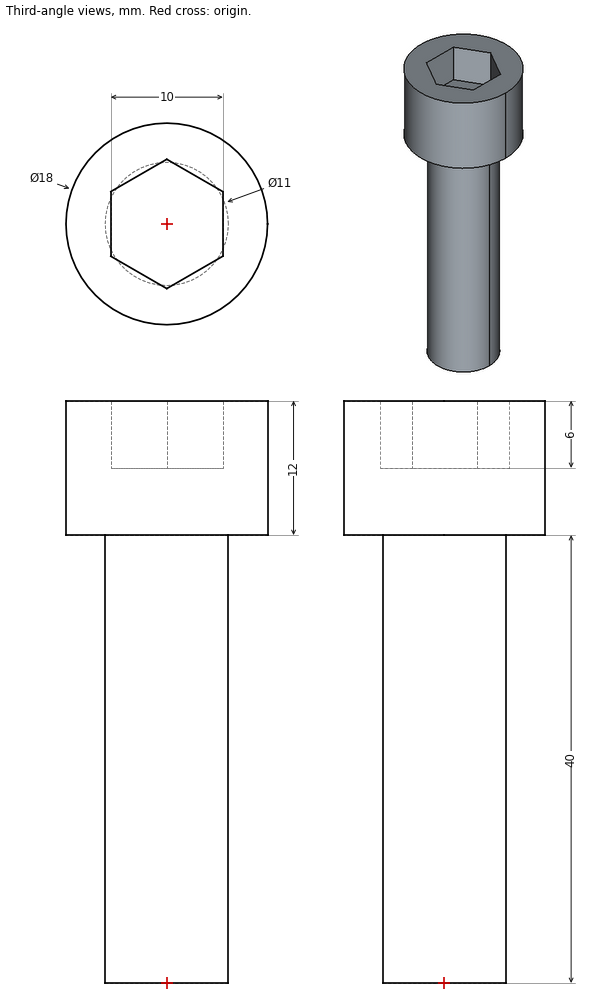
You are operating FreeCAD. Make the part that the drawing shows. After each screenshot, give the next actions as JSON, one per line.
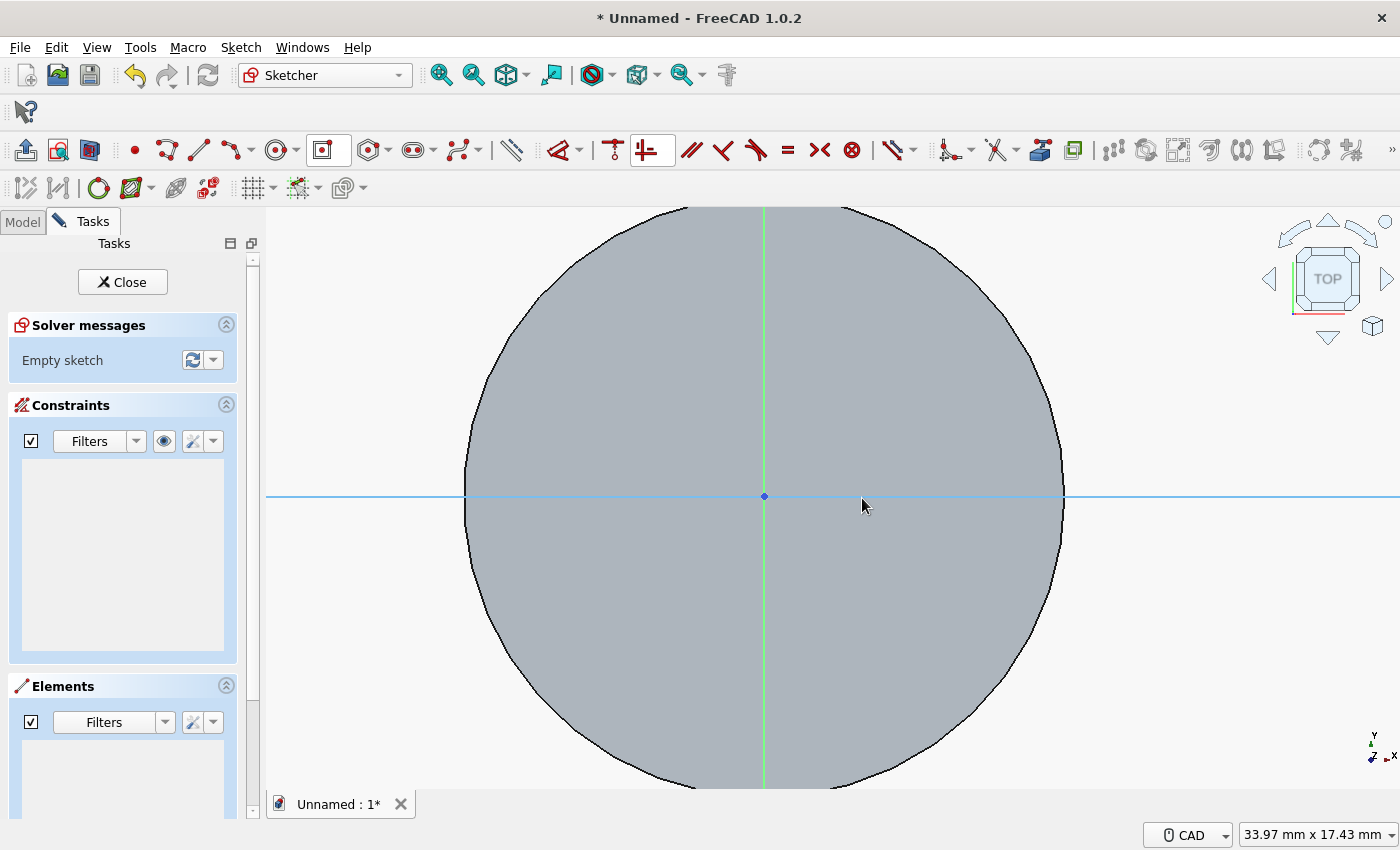
{"action": "left_click", "coordinate": [368, 150]}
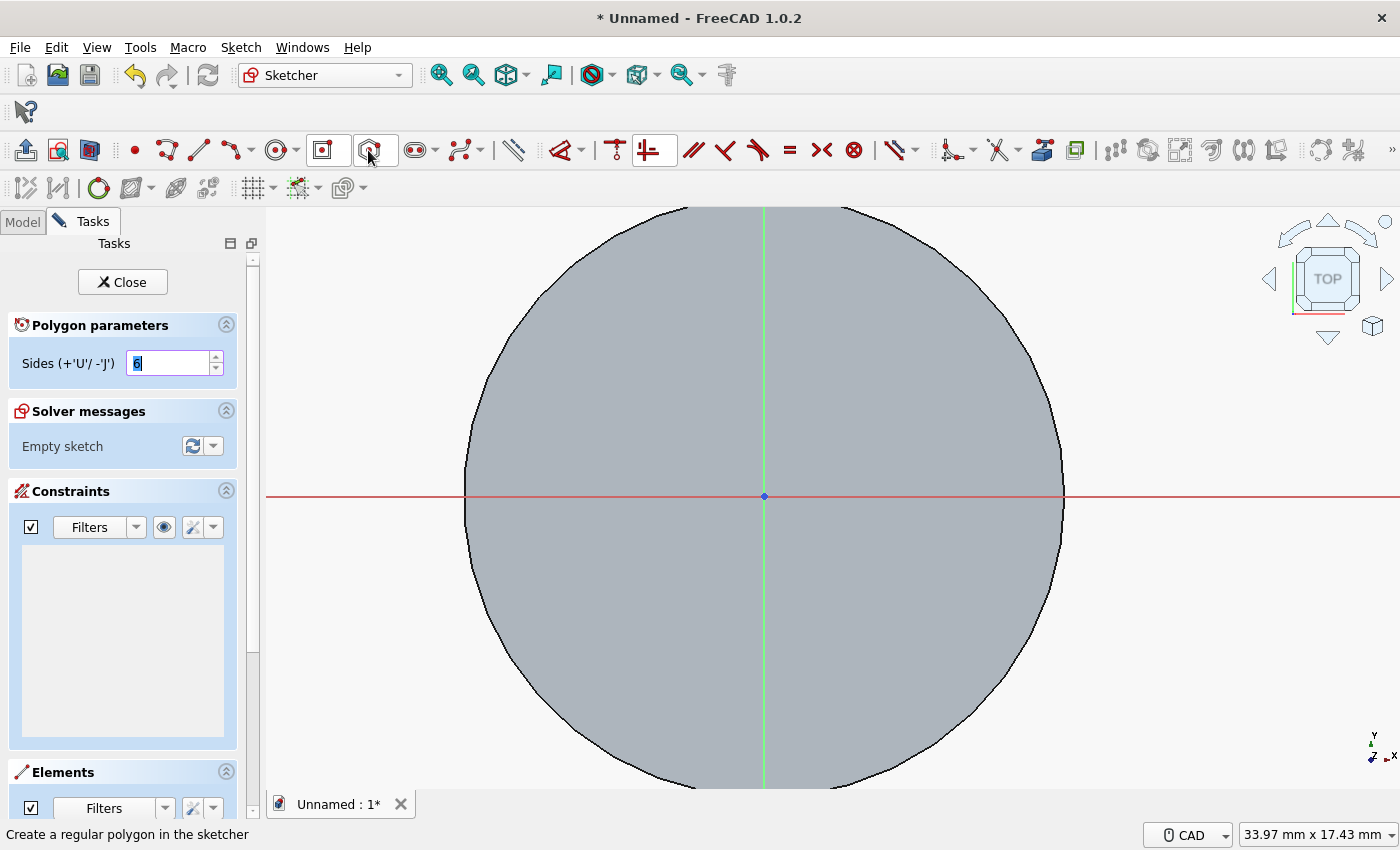
{"action": "left_click", "coordinate": [764, 497]}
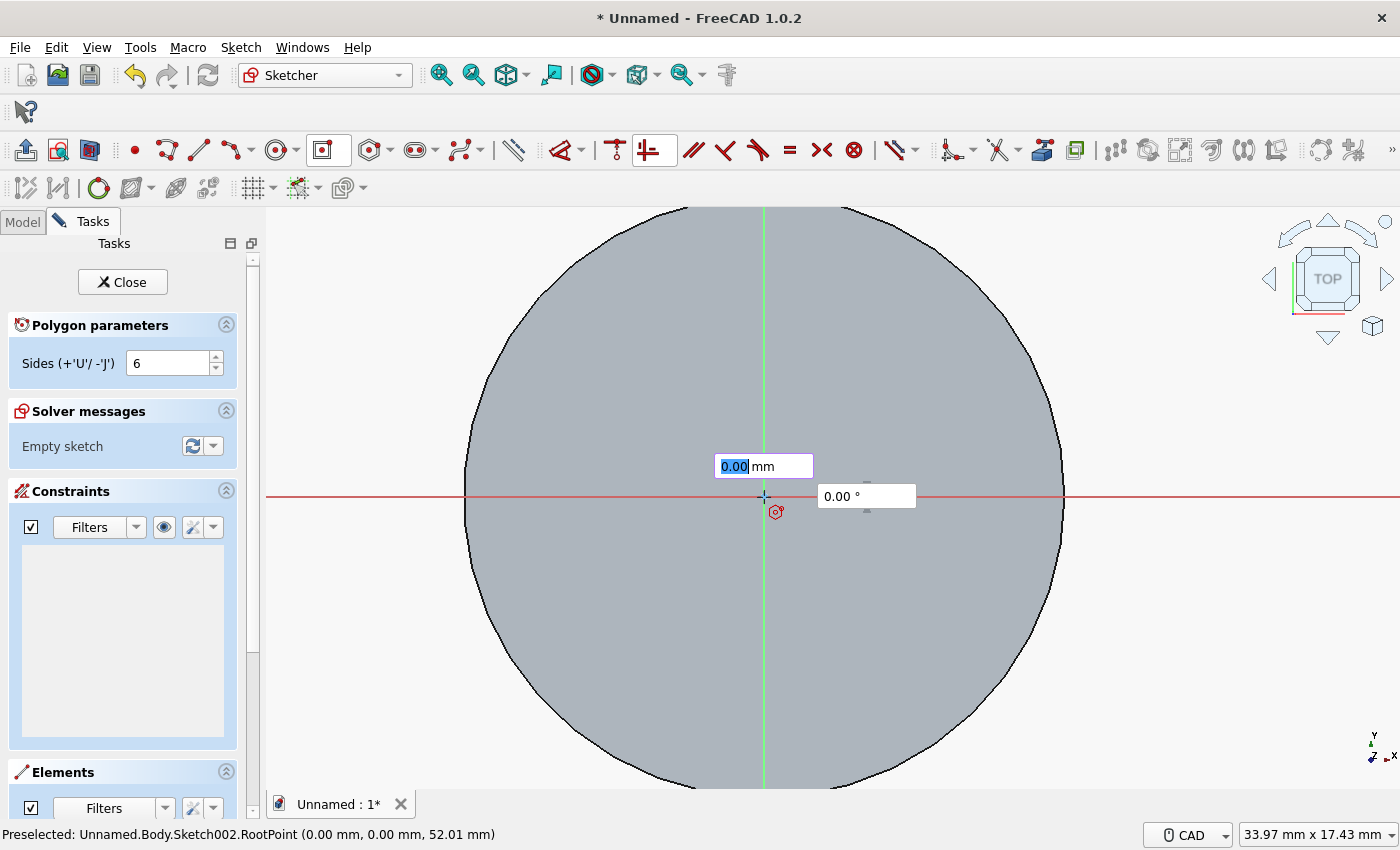
{"action": "left_click", "coordinate": [764, 304]}
{"action": "right_click", "coordinate": [764, 304]}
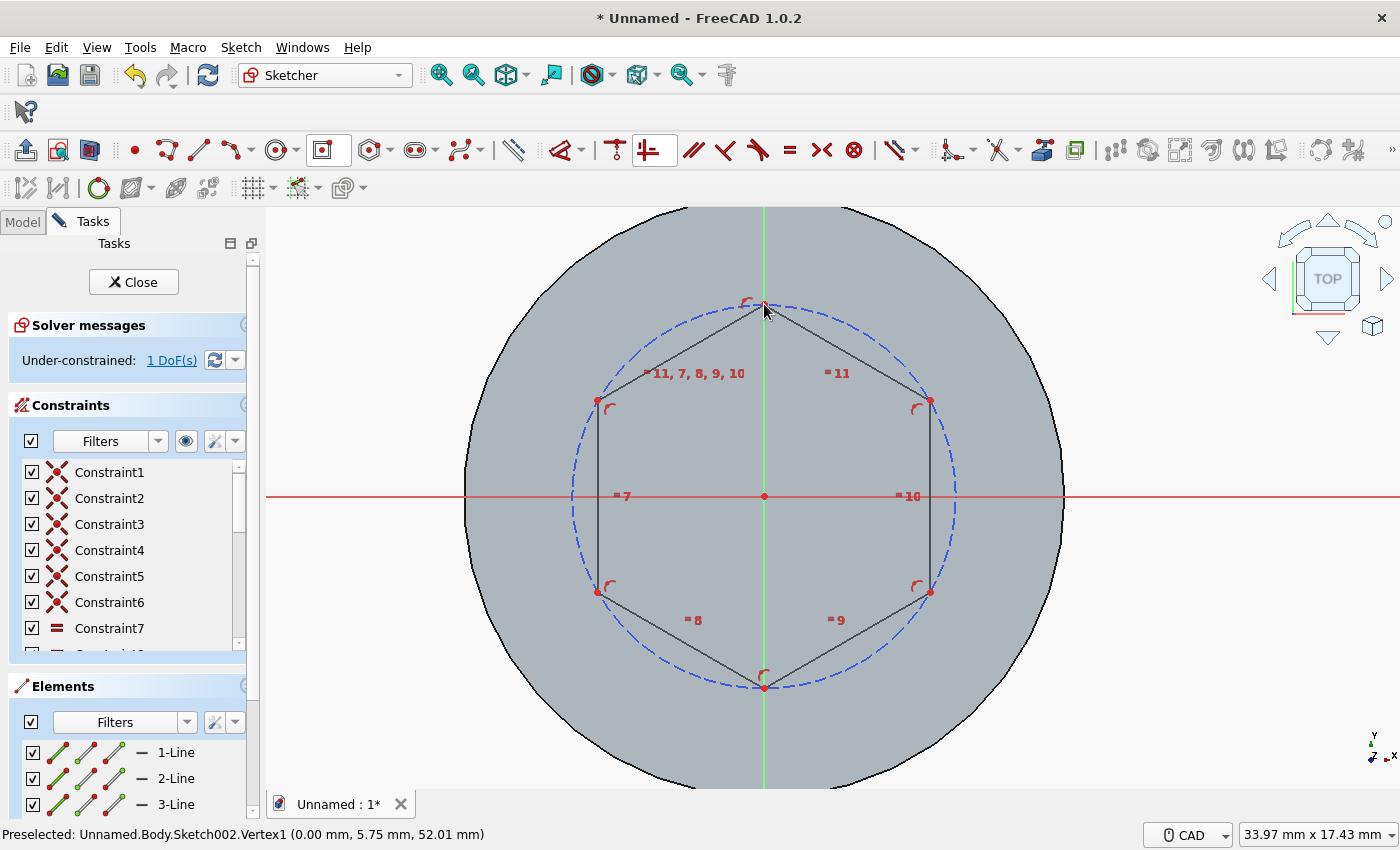
{"action": "left_click", "coordinate": [598, 401]}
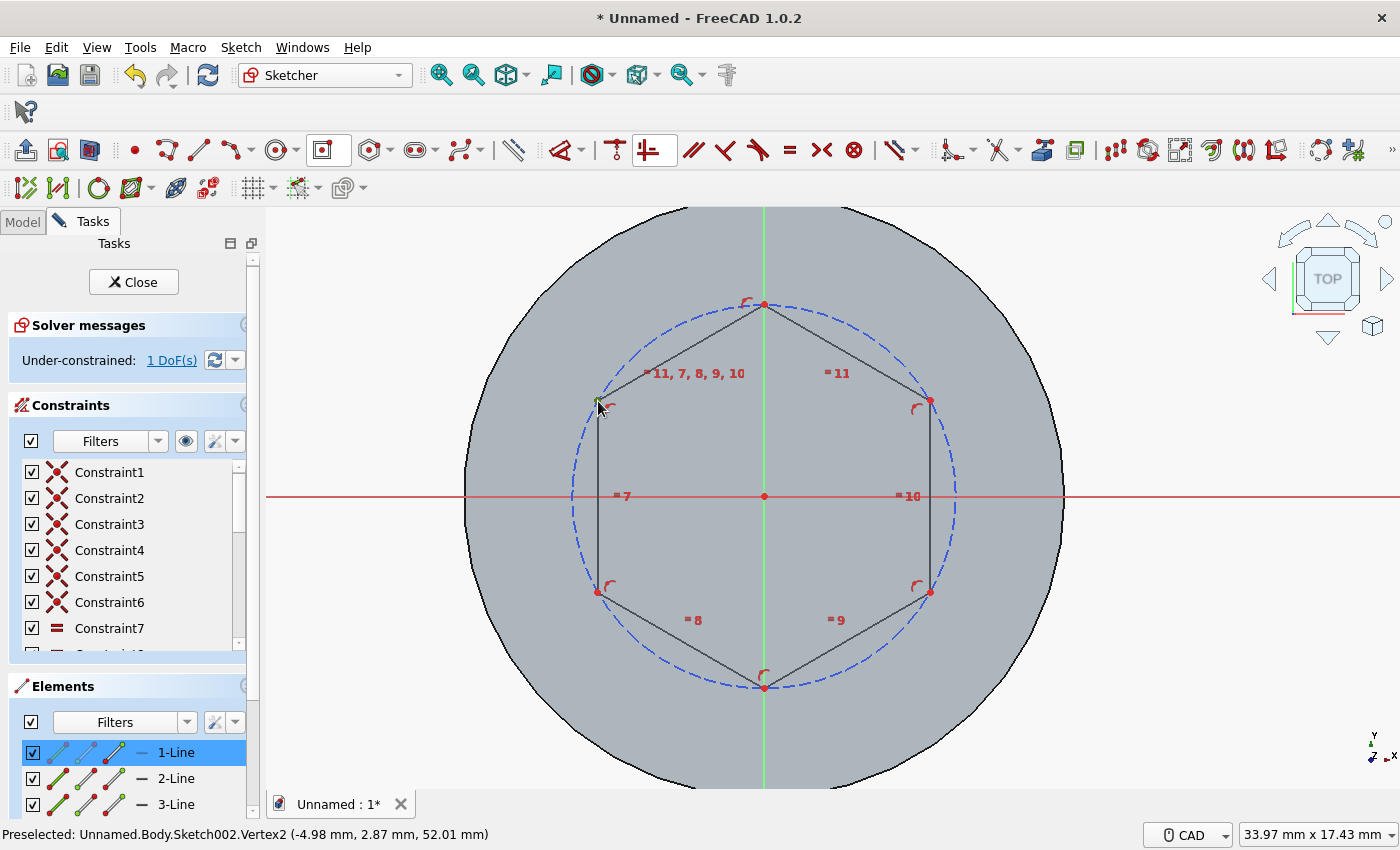
{"action": "left_click", "coordinate": [930, 593]}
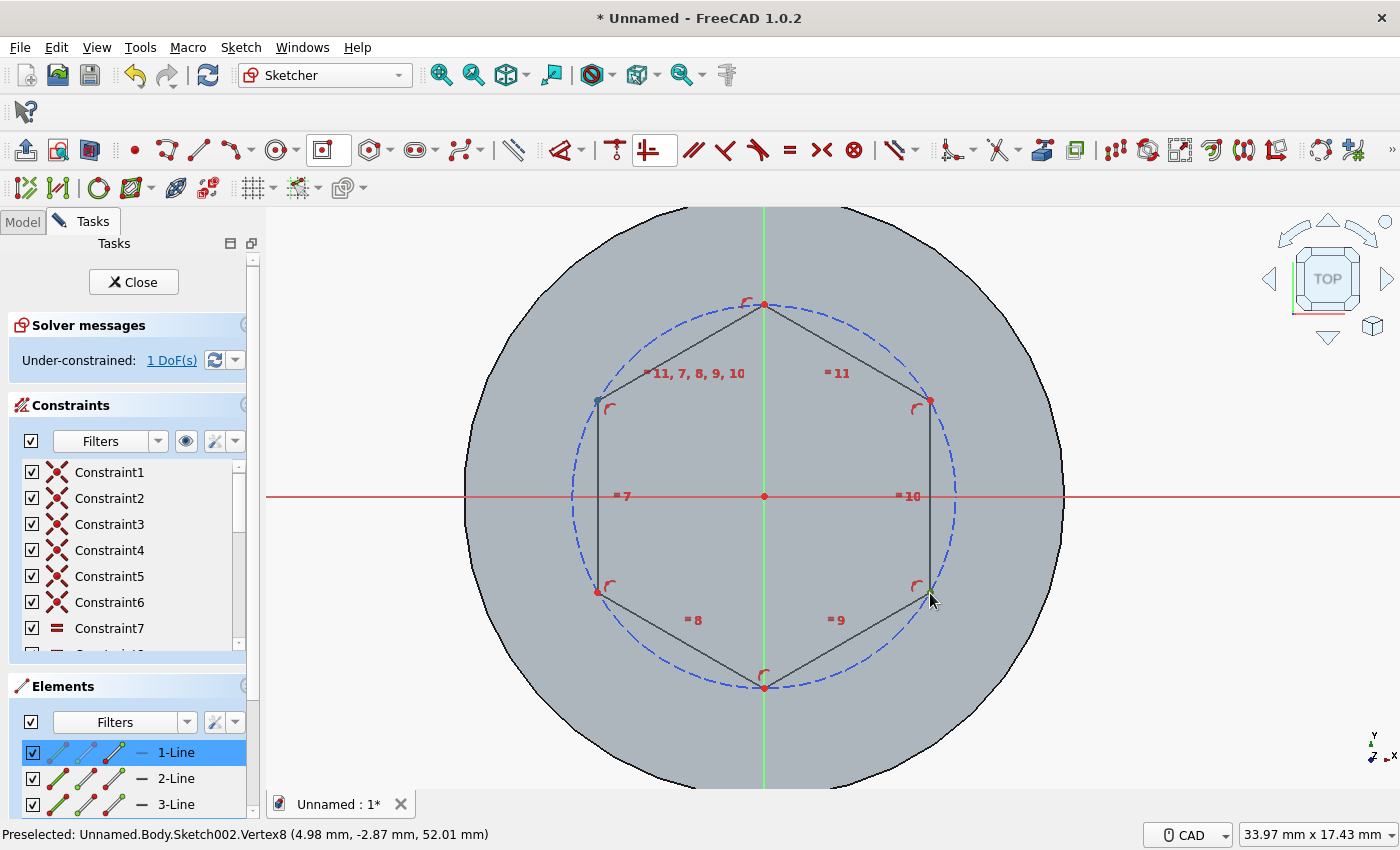
{"action": "key", "text": "l"}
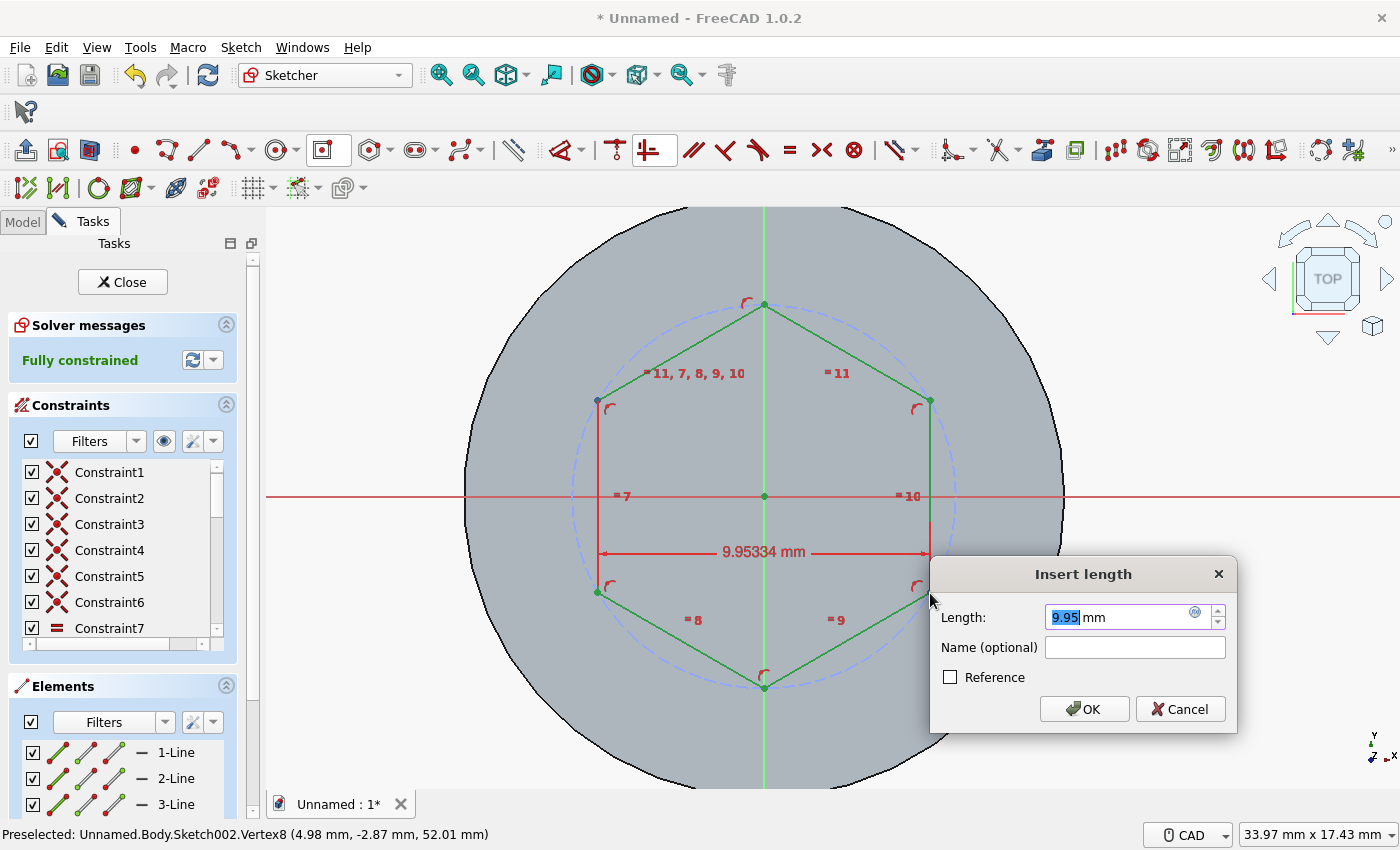
{"action": "type", "text": "10"}
{"action": "key", "text": "Return"}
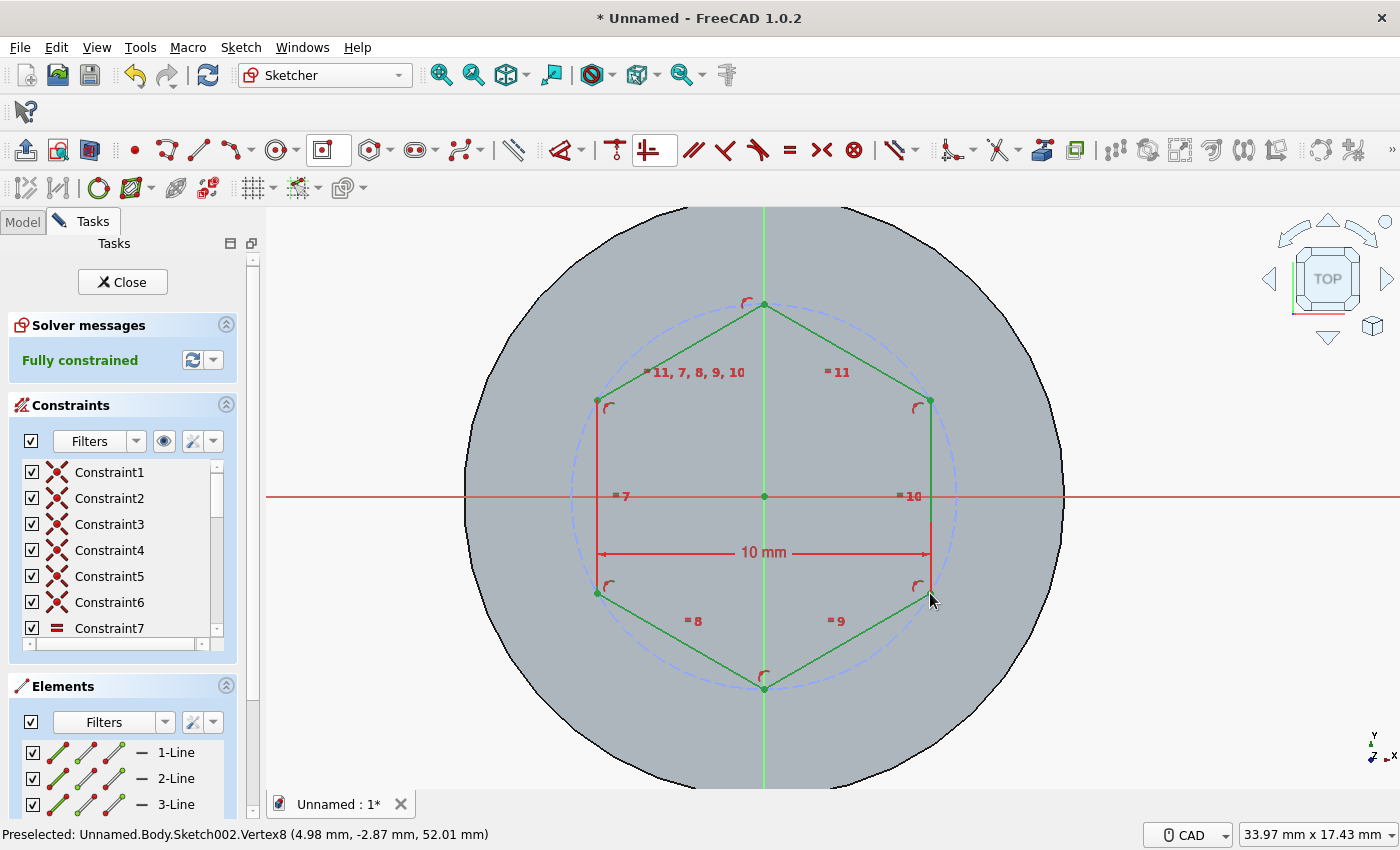
{"action": "left_click", "coordinate": [123, 282]}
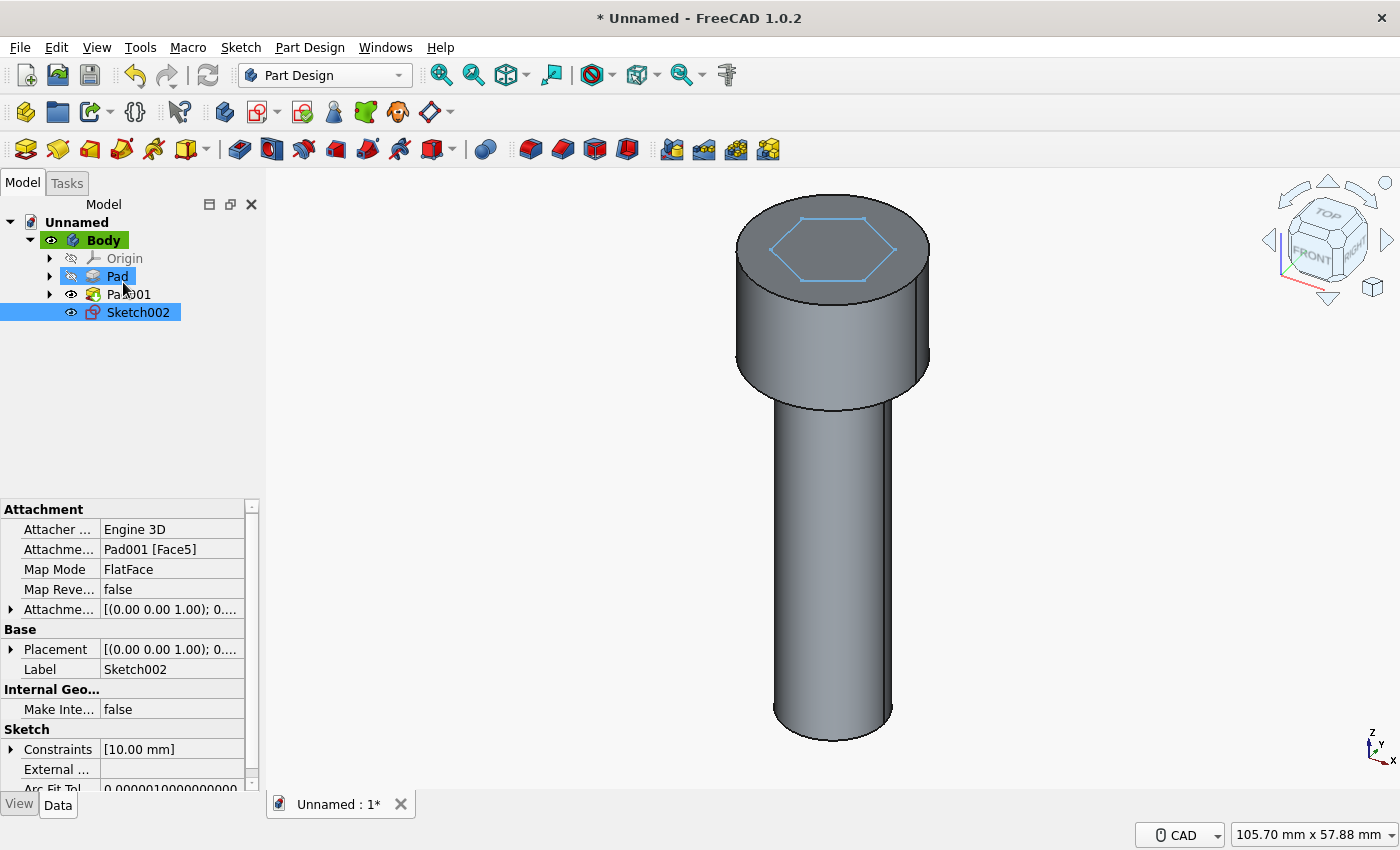
{"action": "left_click", "coordinate": [240, 150]}